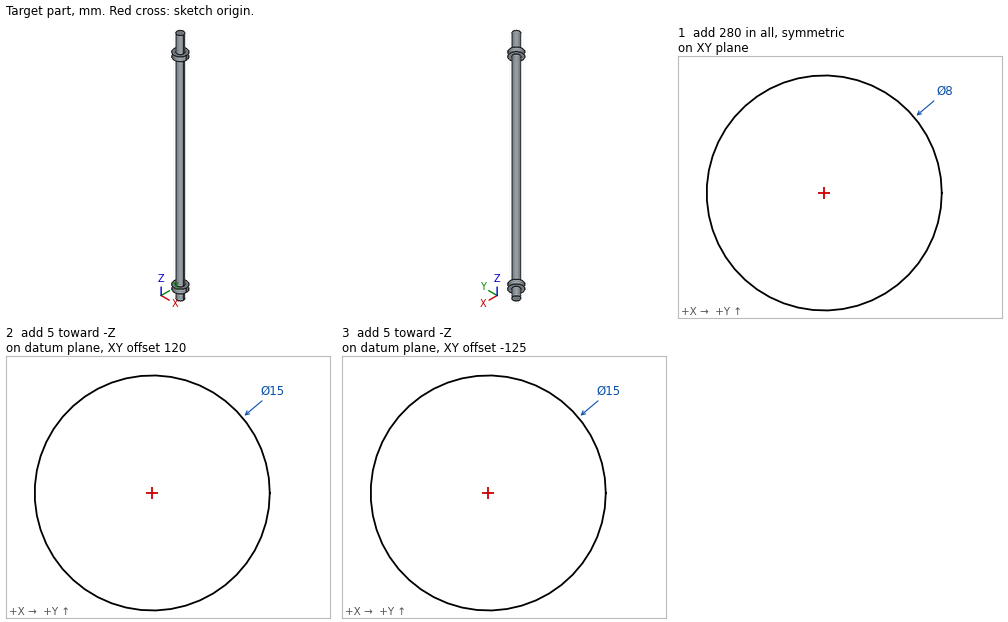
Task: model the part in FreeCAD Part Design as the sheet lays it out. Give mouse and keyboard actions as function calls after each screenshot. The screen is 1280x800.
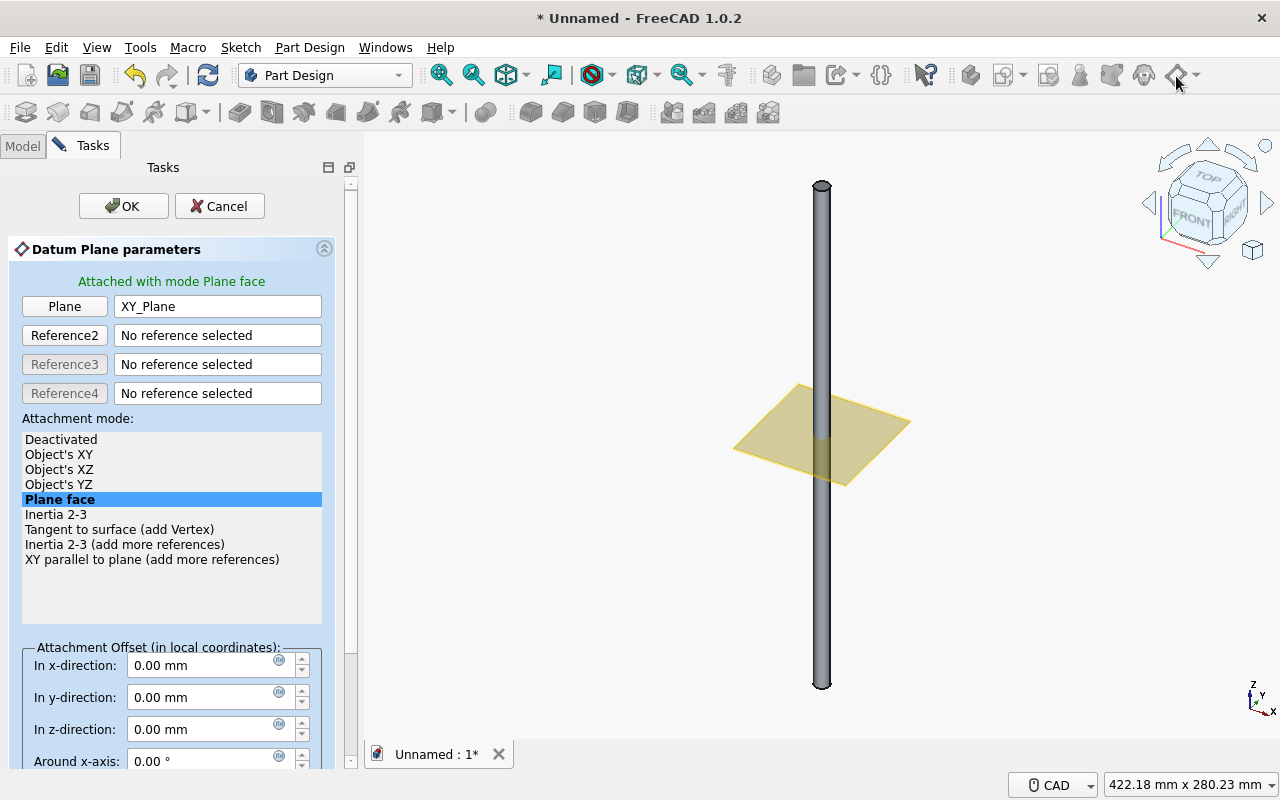
triple_click(210, 729)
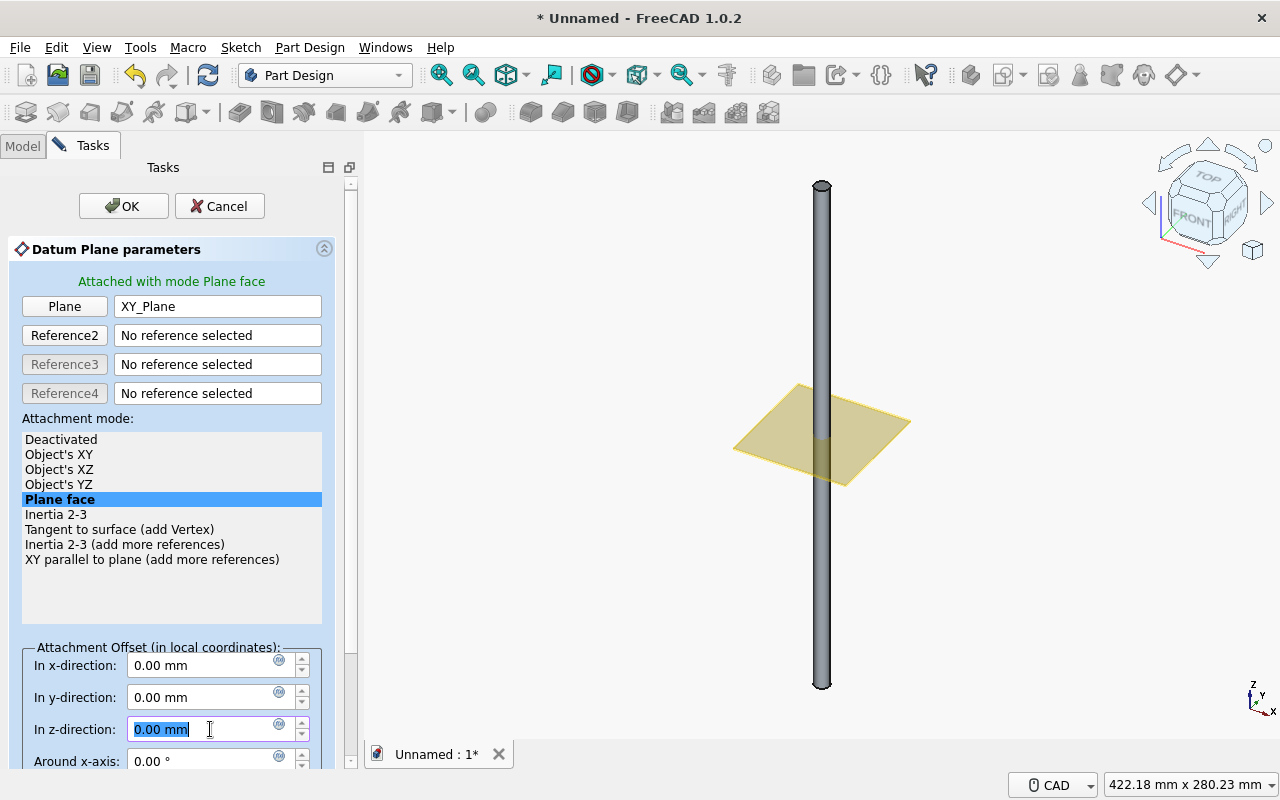
text(120)
key(Tab)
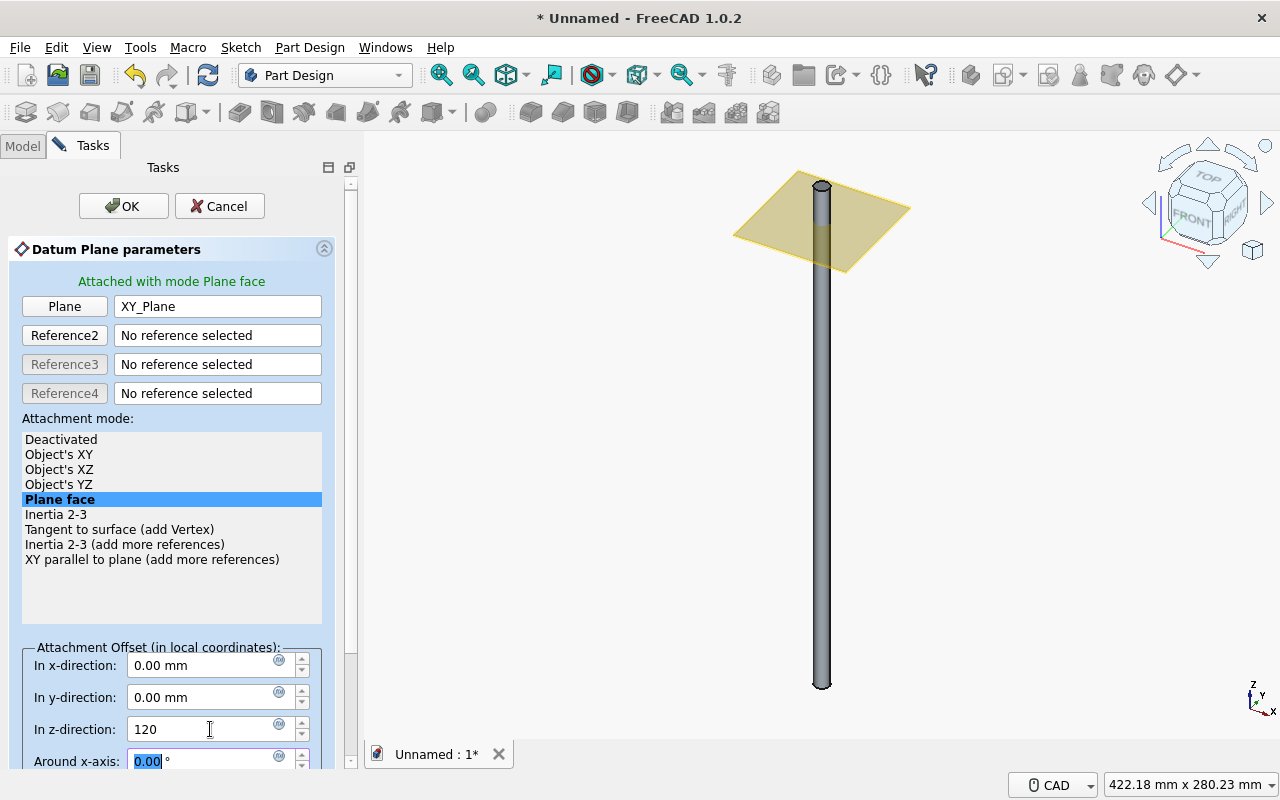
click(124, 206)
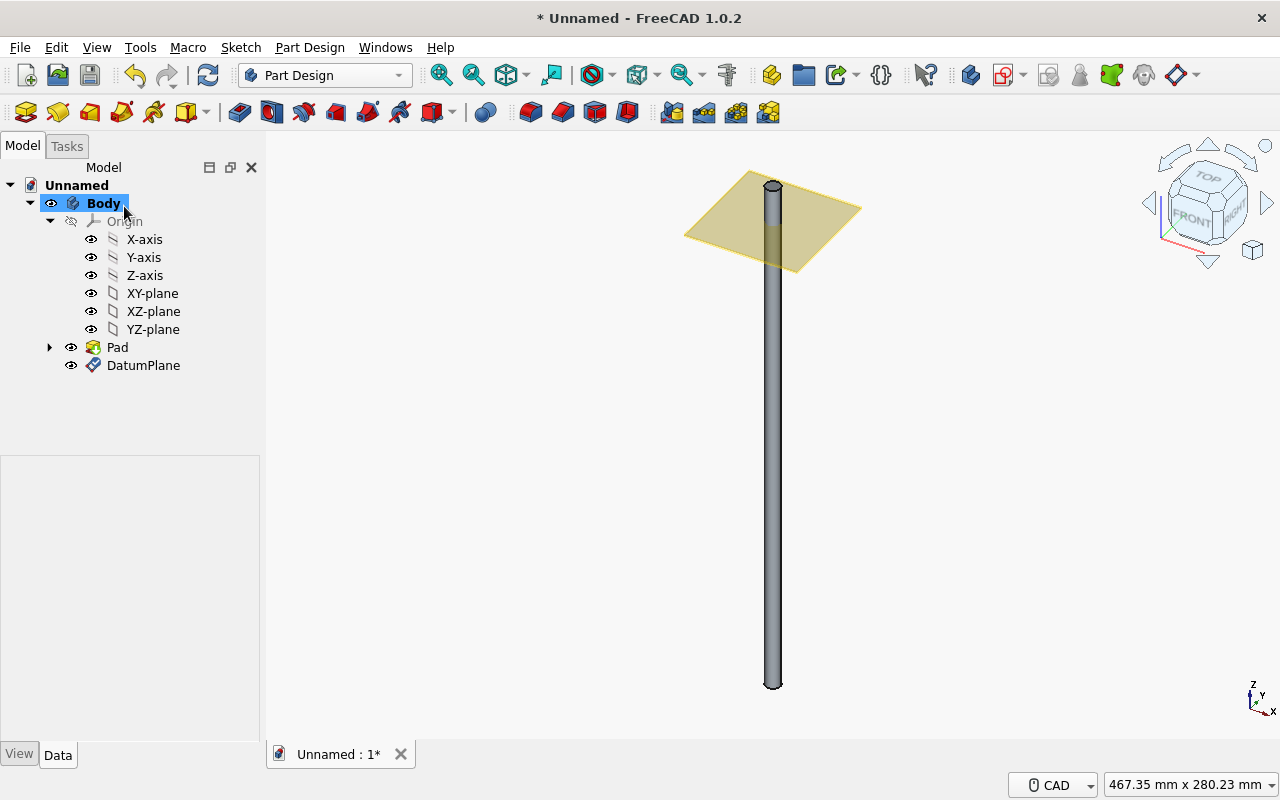
click(116, 365)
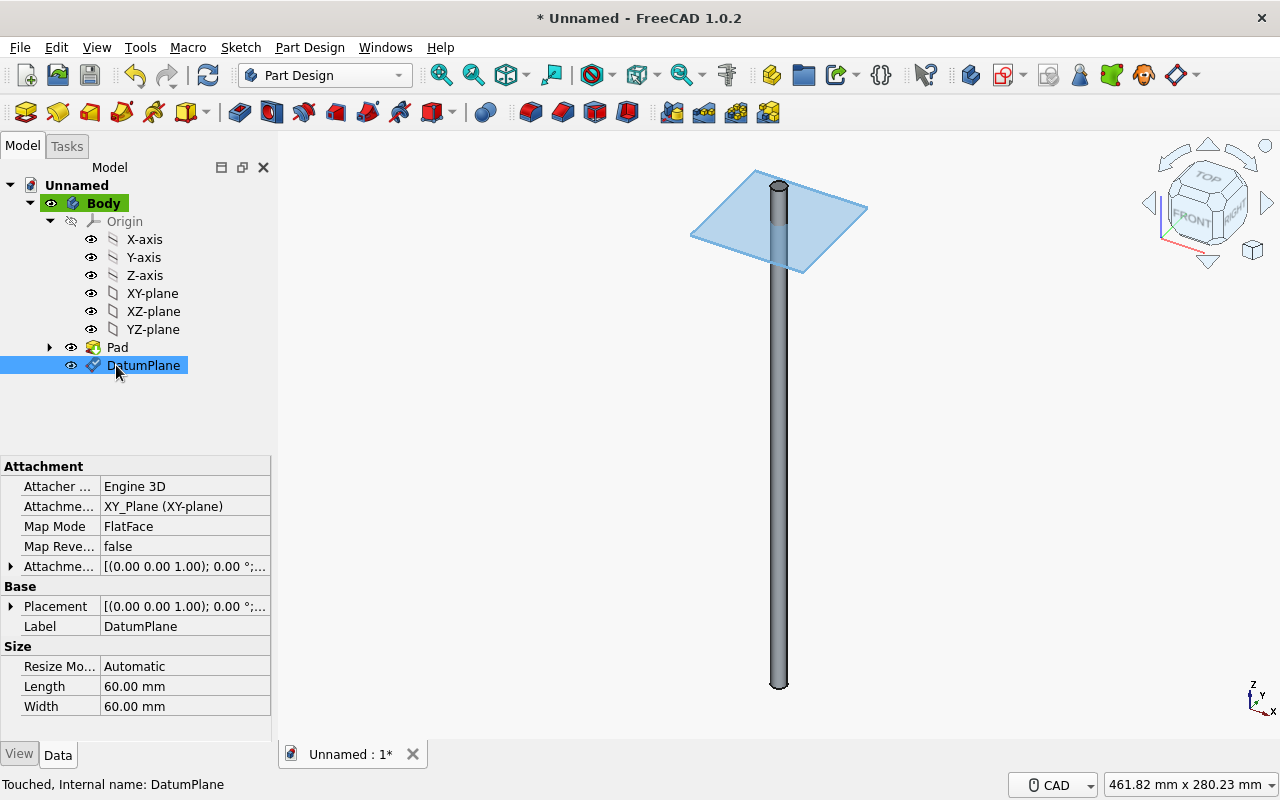
click(1004, 76)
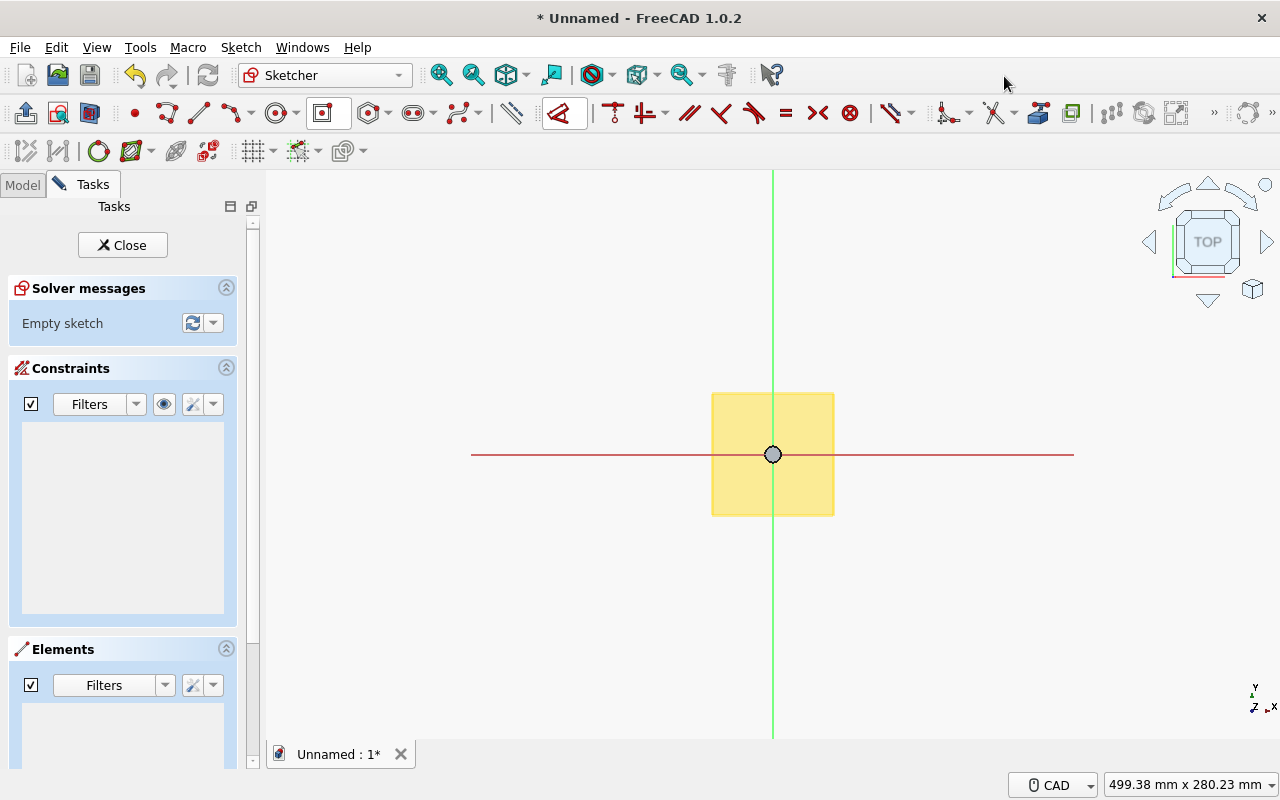
key(q)
key(s)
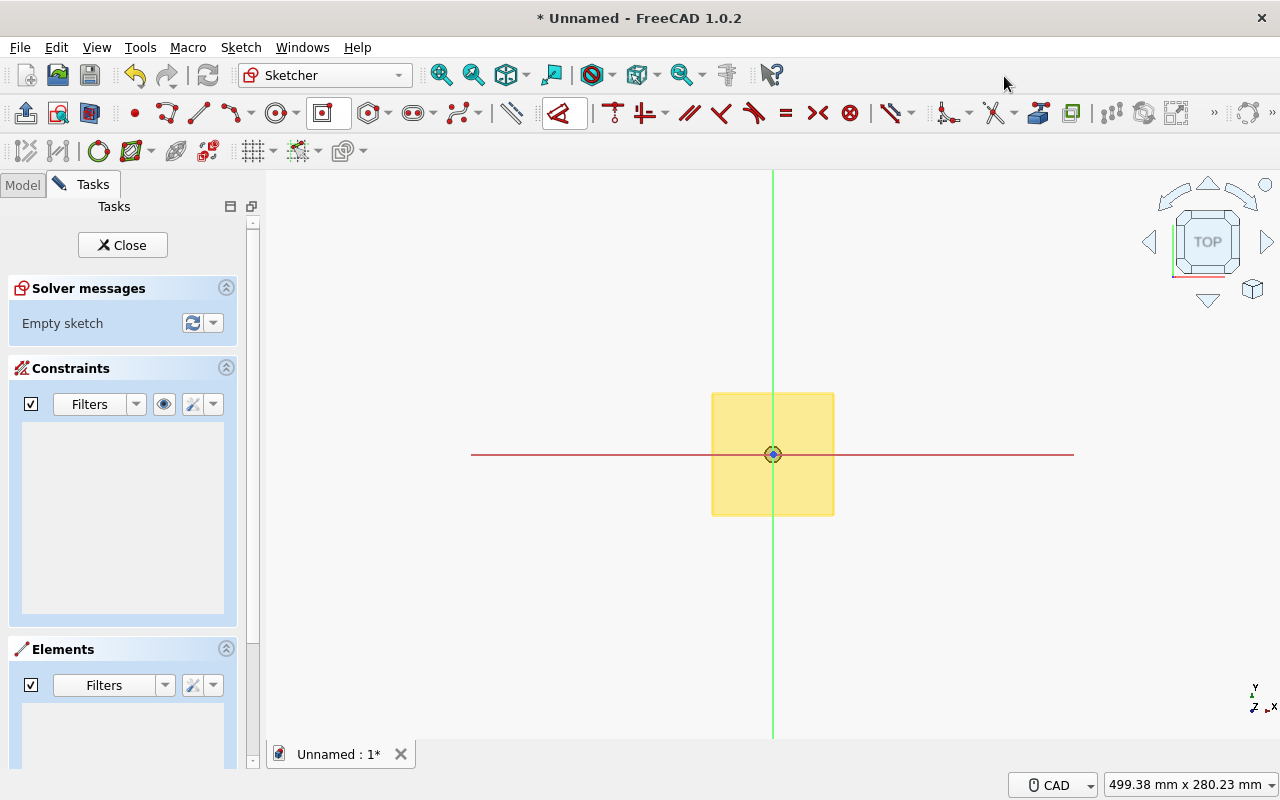
scroll(780, 455, up, 12)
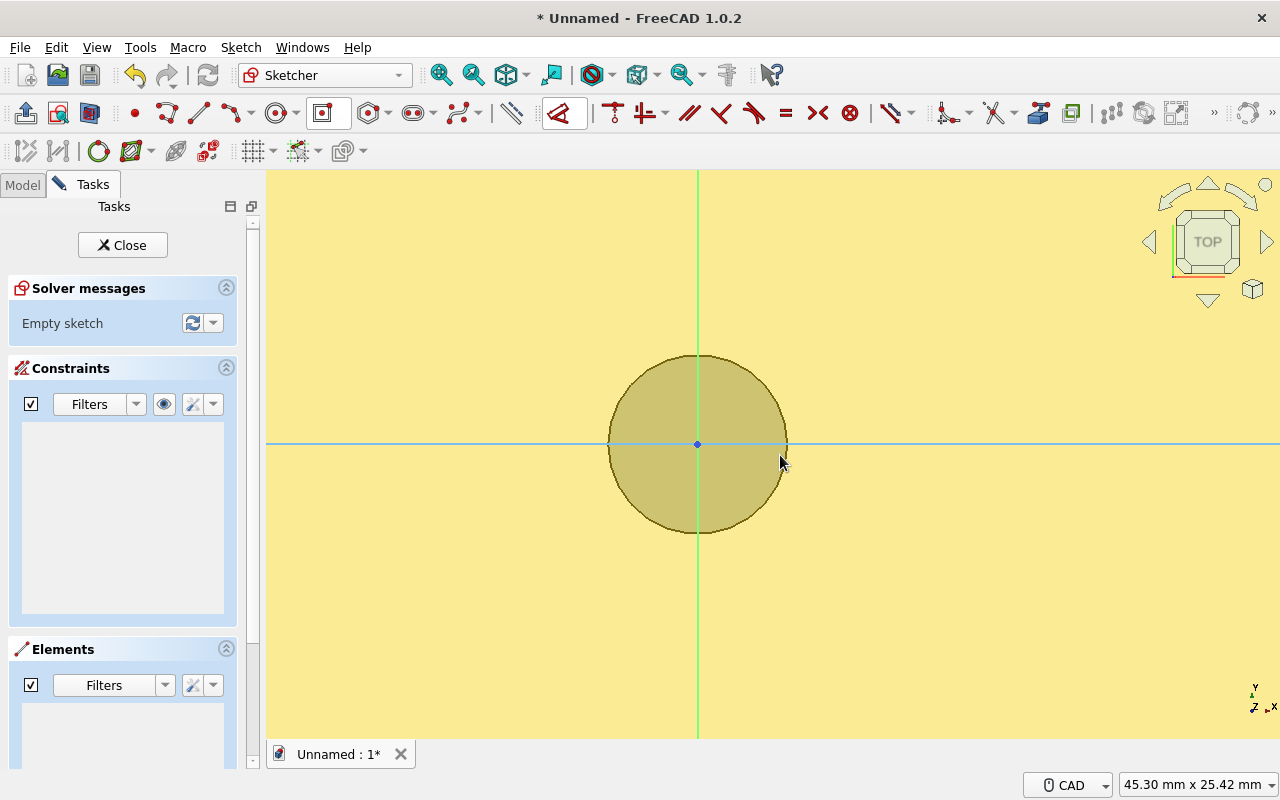
key(g)
key(c)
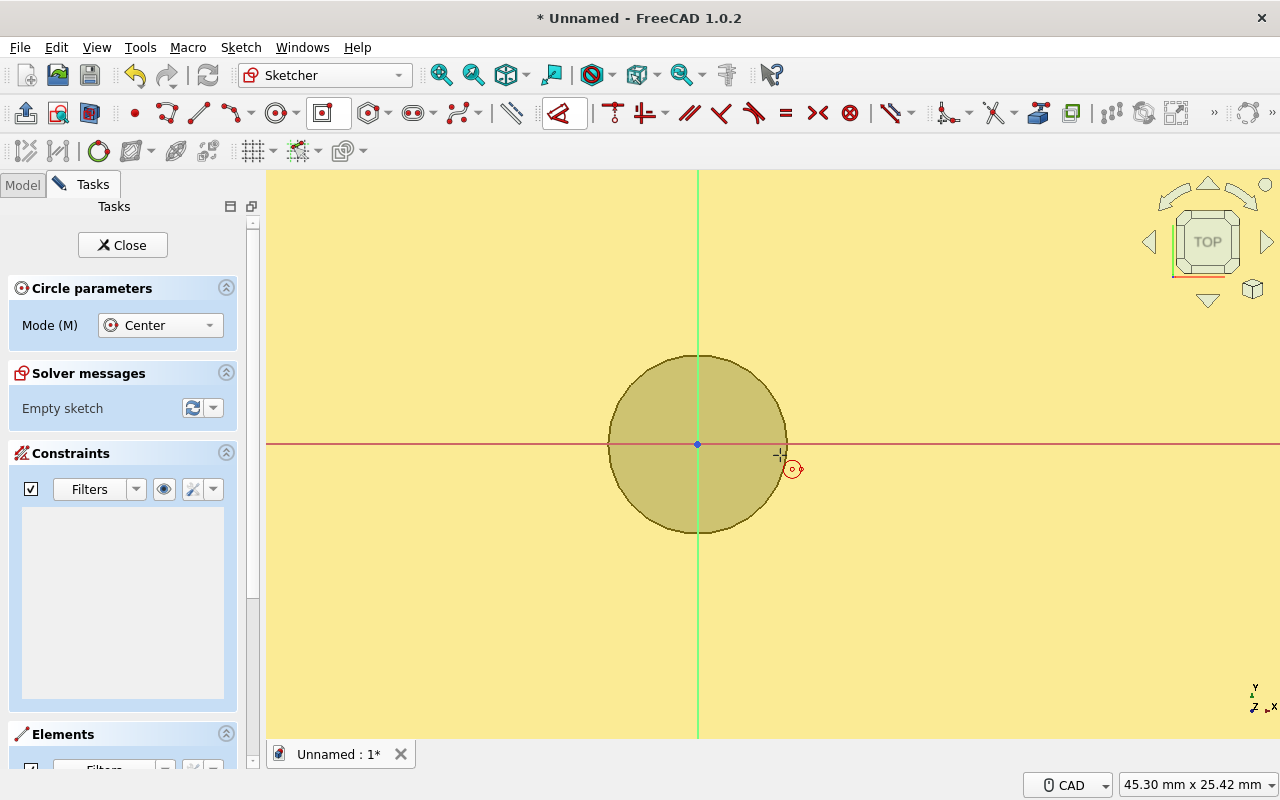
click(698, 444)
click(816, 326)
key(Escape)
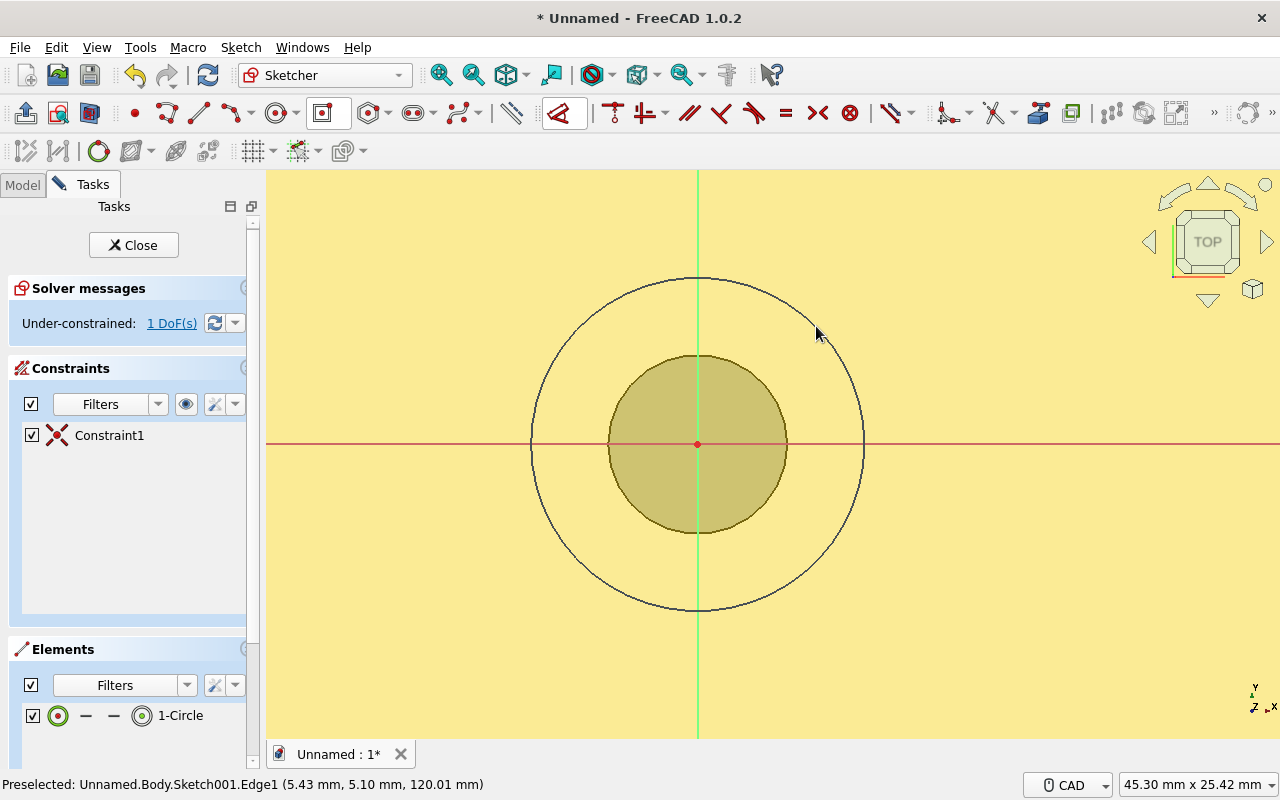
click(815, 326)